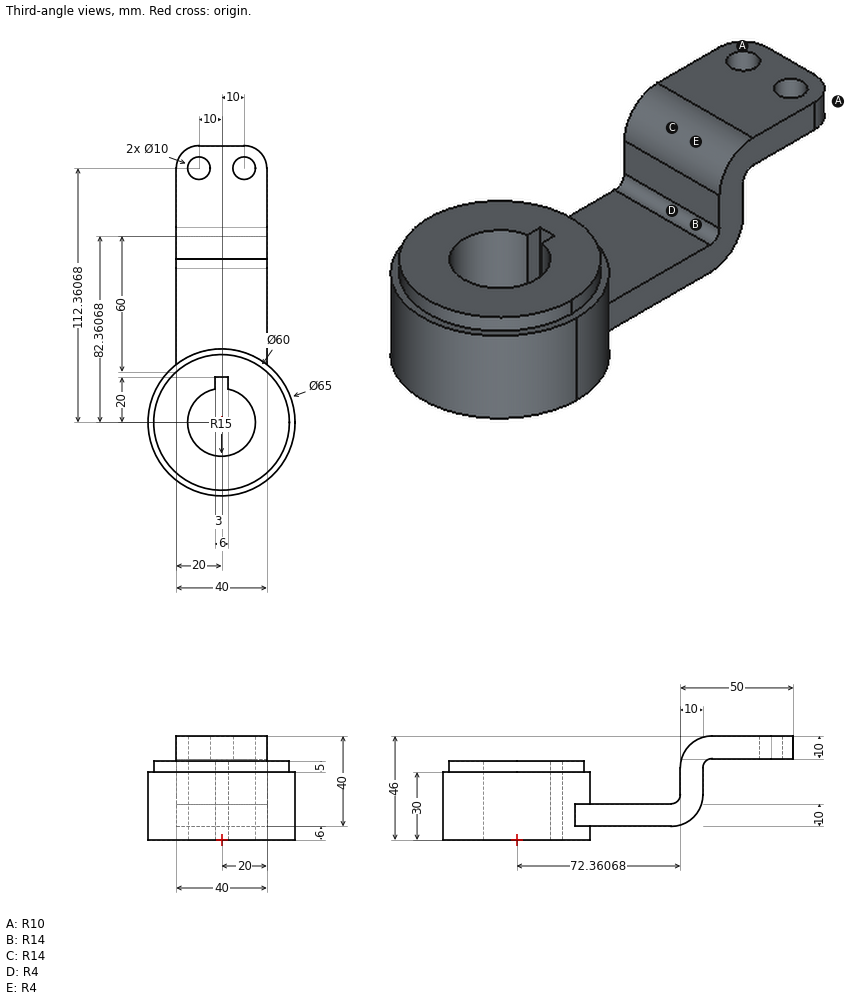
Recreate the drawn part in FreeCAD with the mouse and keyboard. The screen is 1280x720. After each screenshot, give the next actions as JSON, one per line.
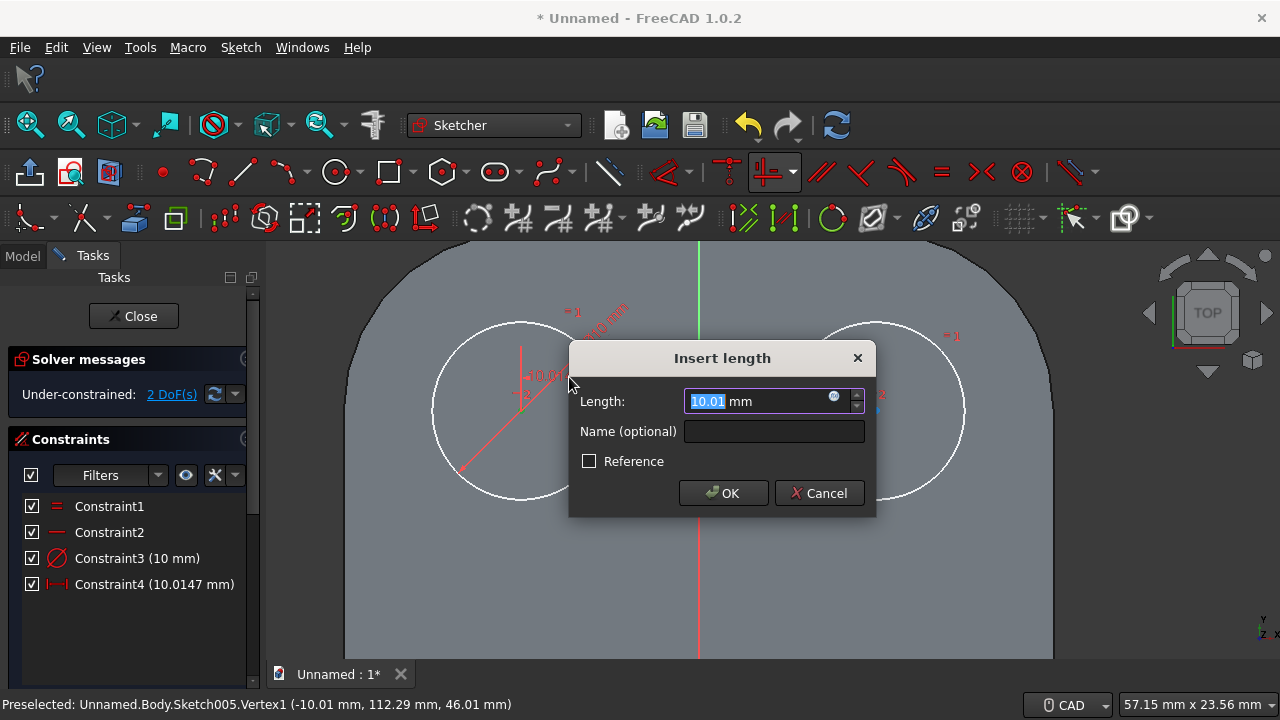
{"action": "type", "text": "10"}
{"action": "key", "text": "Return"}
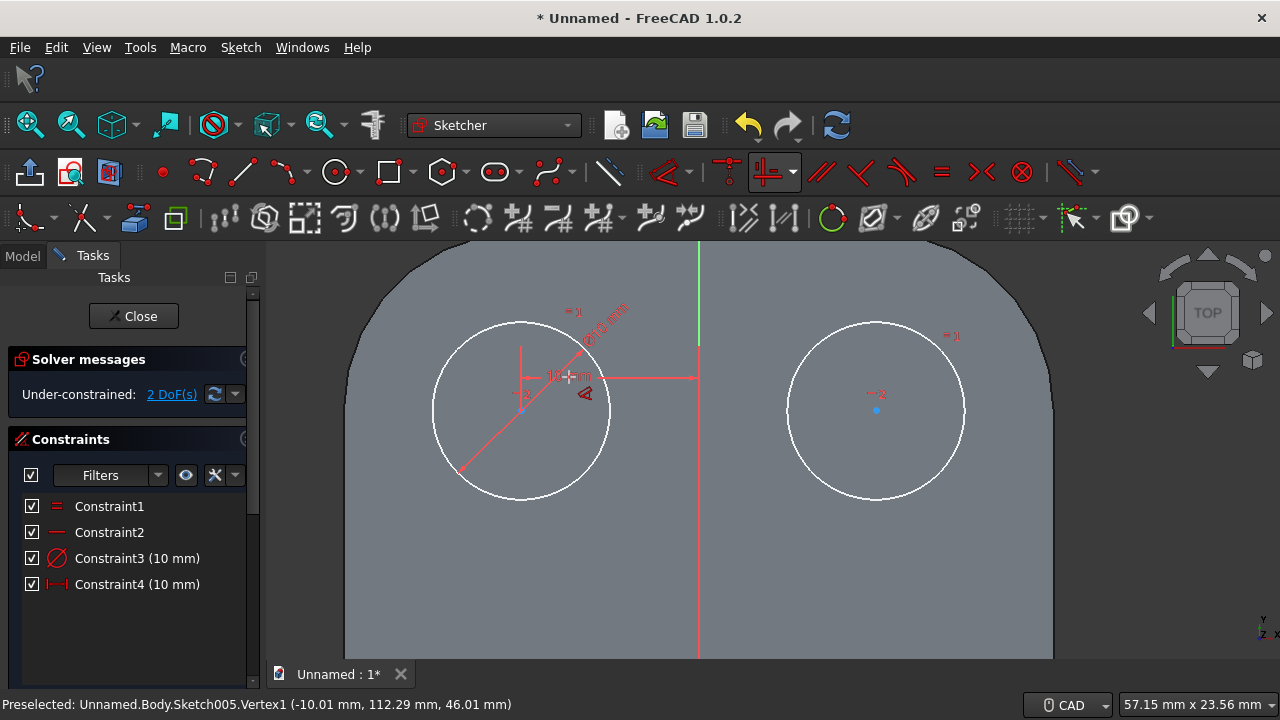
{"action": "left_click", "coordinate": [876, 411]}
{"action": "left_click", "coordinate": [747, 377]}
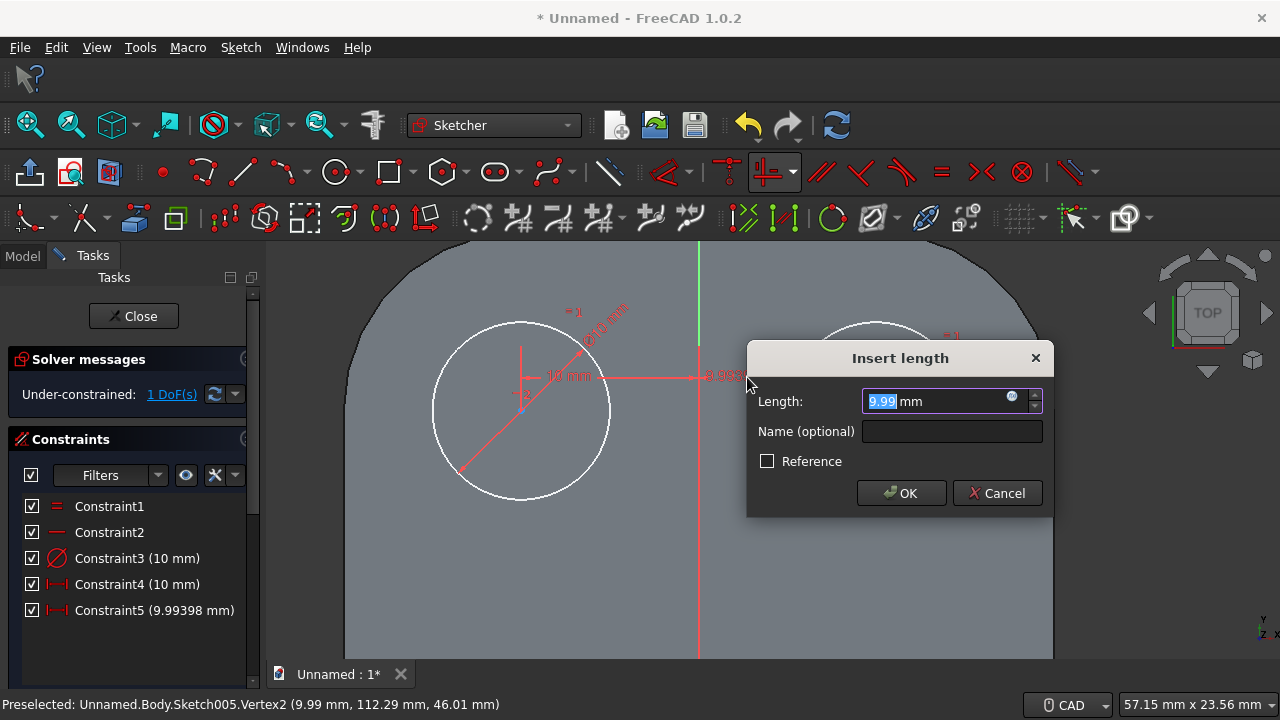
{"action": "type", "text": "10"}
{"action": "key", "text": "Return"}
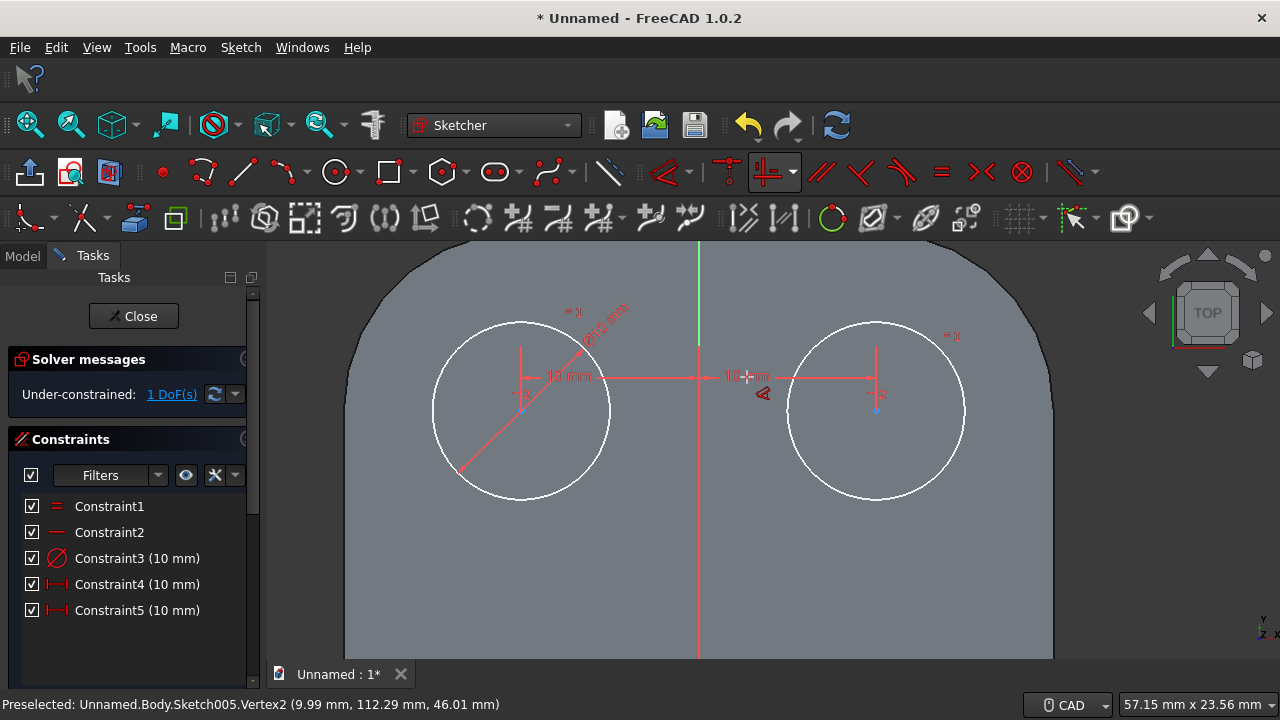
{"action": "left_click", "coordinate": [521, 411]}
{"action": "left_click", "coordinate": [487, 521]}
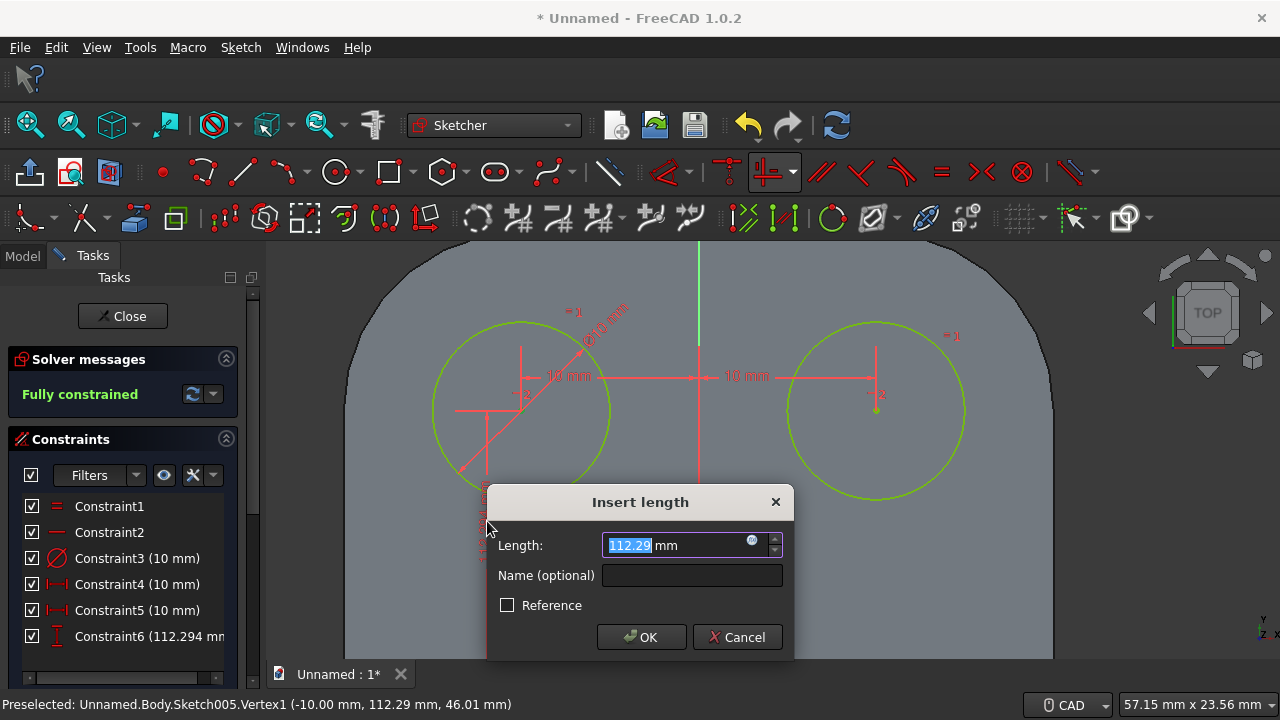
{"action": "type", "text": "112.36068"}
{"action": "key", "text": "Return"}
{"action": "key", "text": "Escape"}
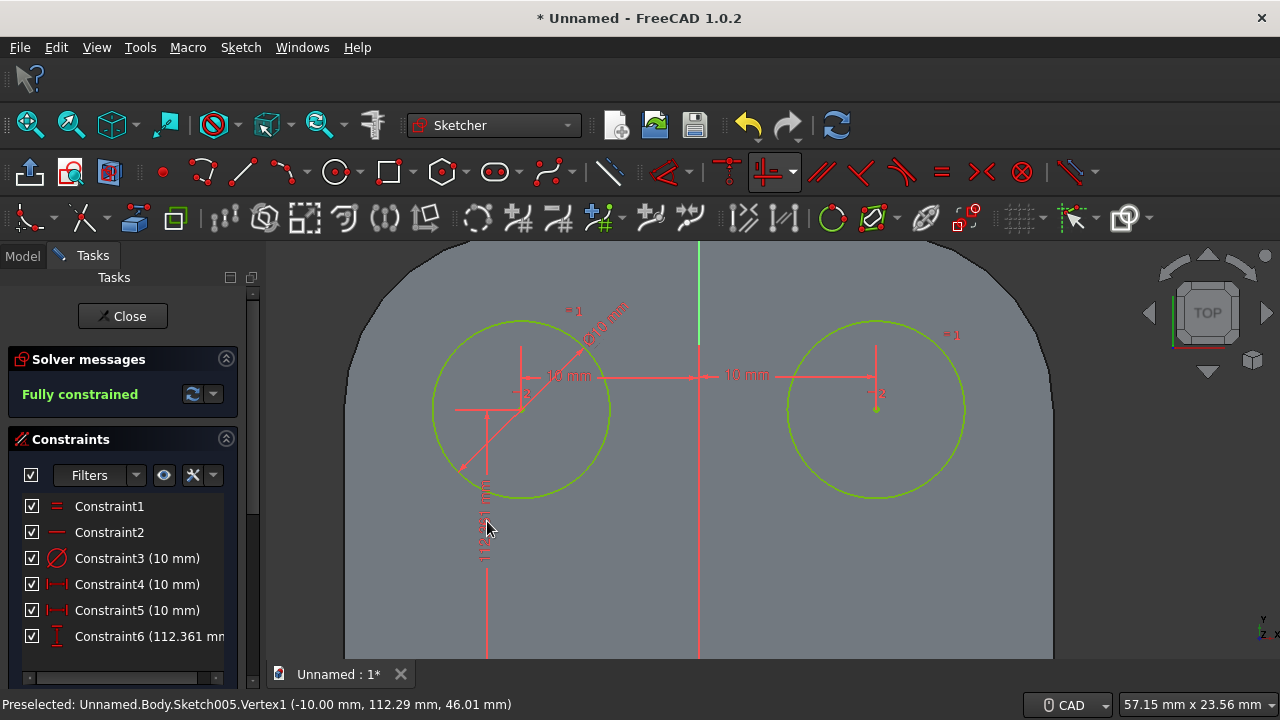
{"action": "left_click", "coordinate": [123, 316]}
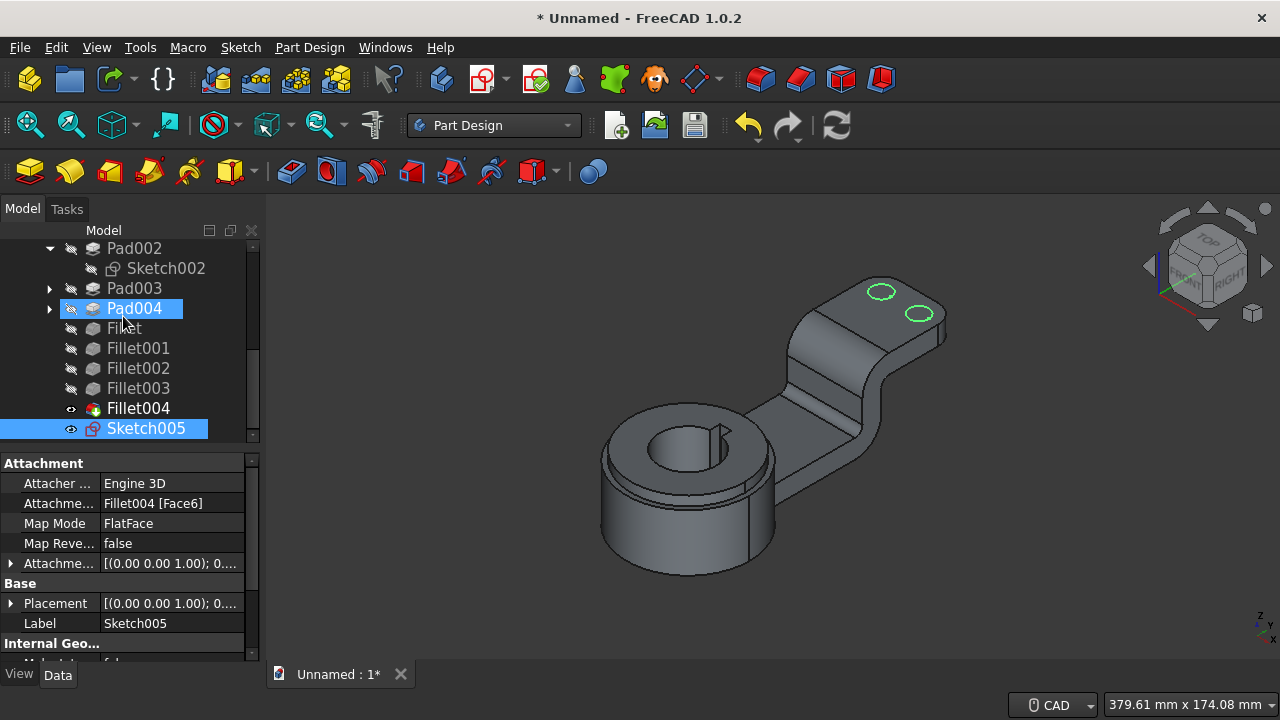
{"action": "left_click", "coordinate": [292, 172]}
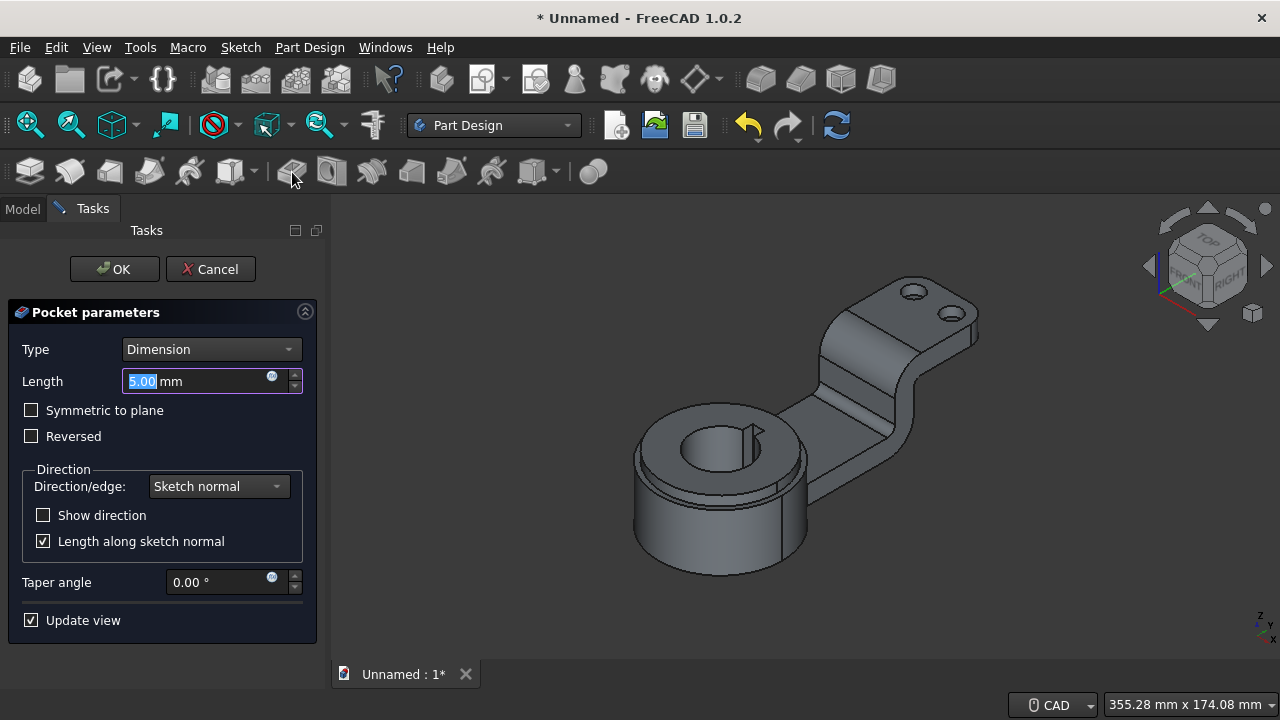
{"action": "type", "text": "40"}
{"action": "key", "text": "Tab"}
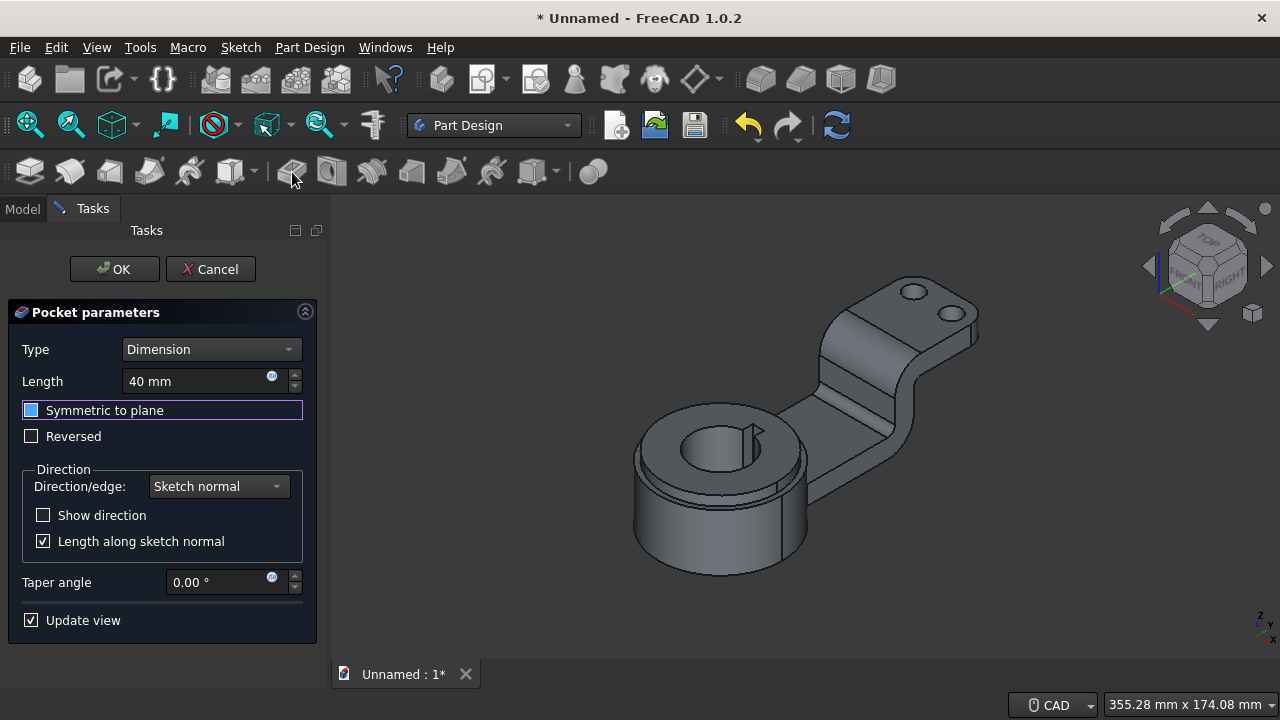
{"action": "left_click", "coordinate": [115, 269]}